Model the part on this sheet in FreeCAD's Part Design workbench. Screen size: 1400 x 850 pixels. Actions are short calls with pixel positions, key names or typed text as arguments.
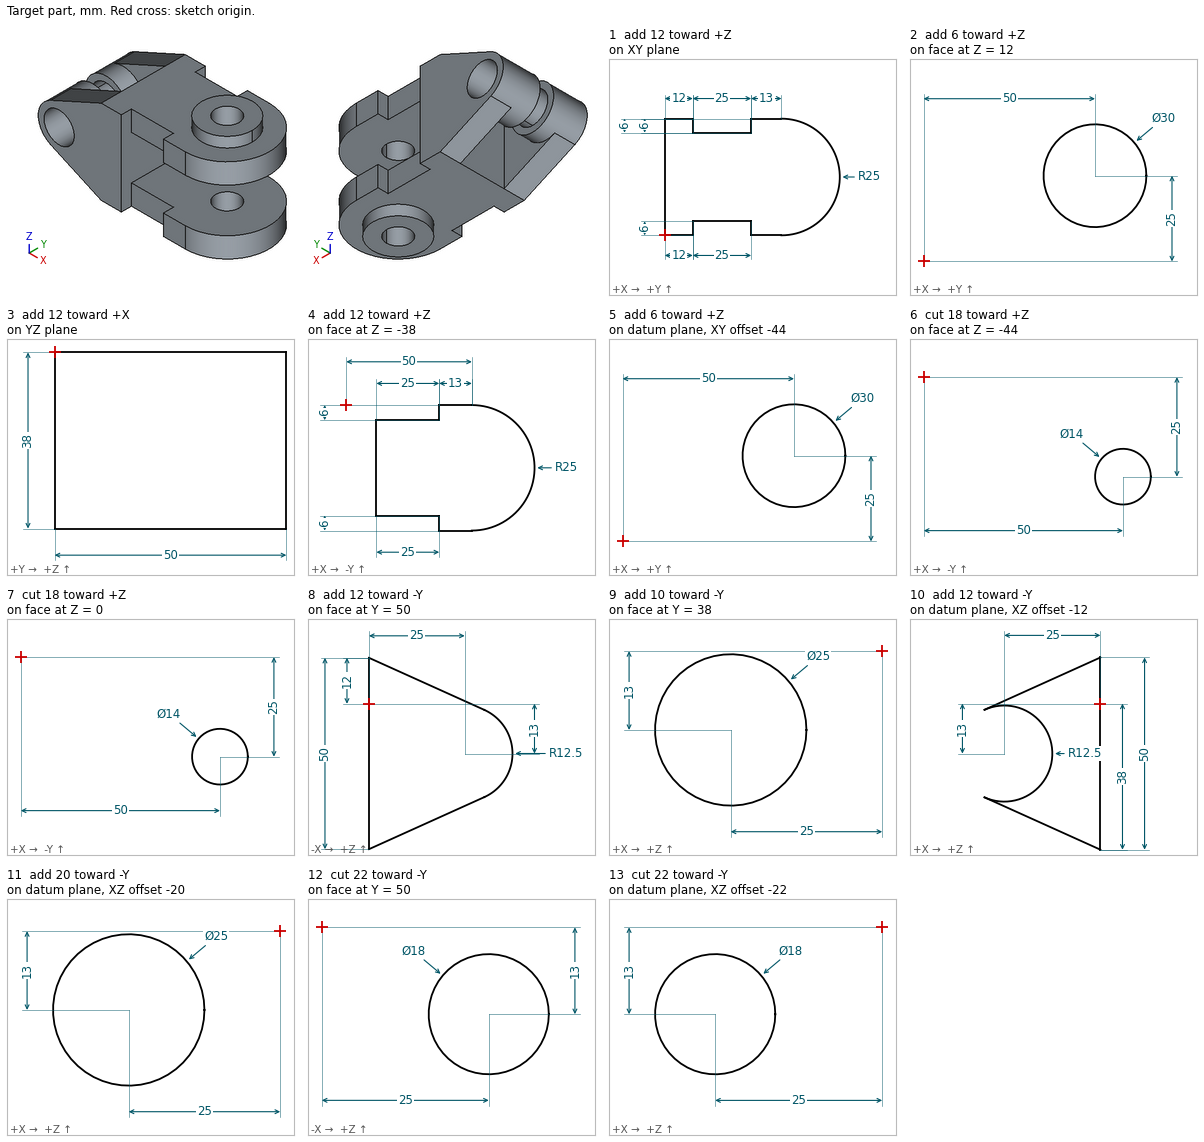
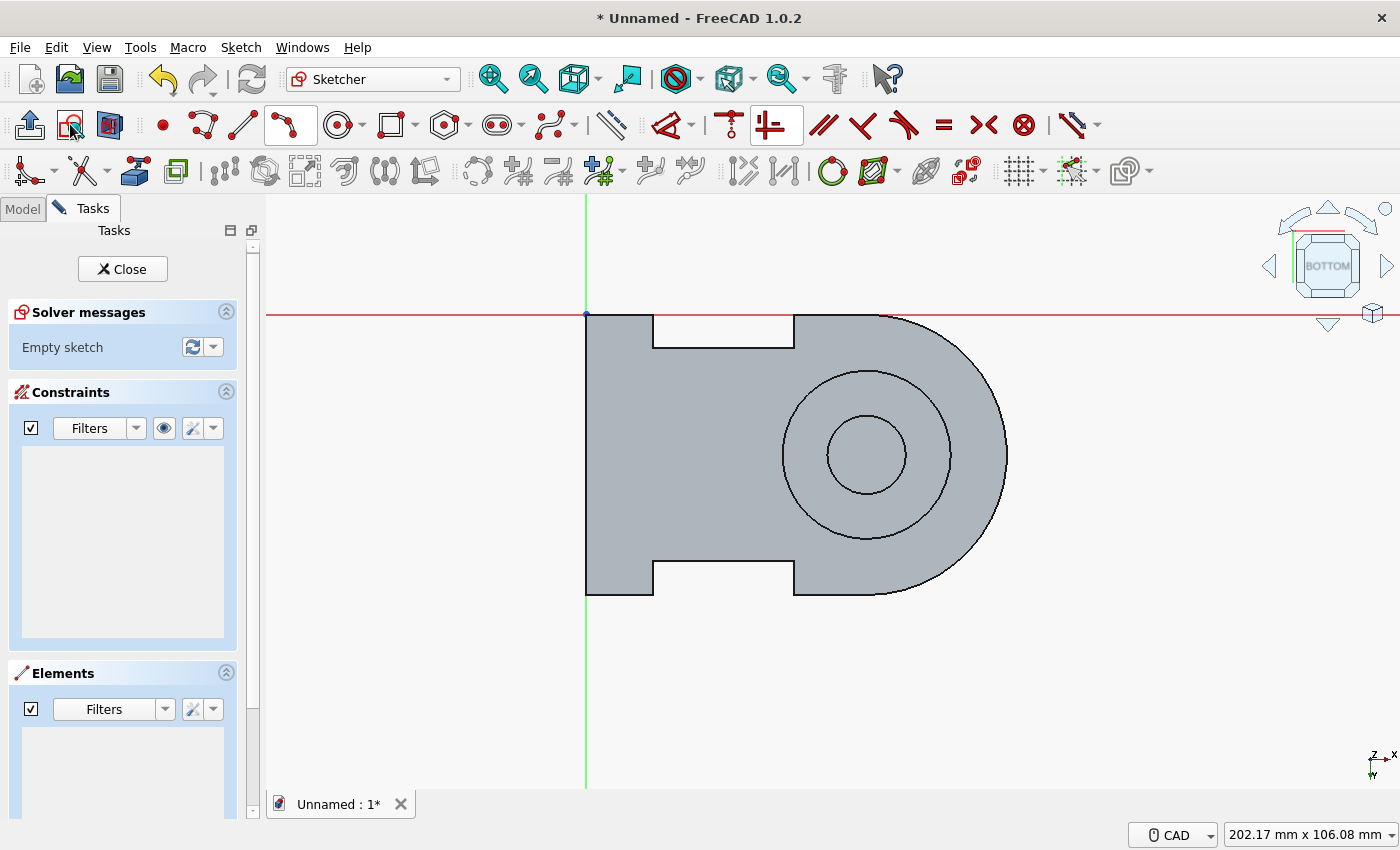
scroll(892, 446, up, 8)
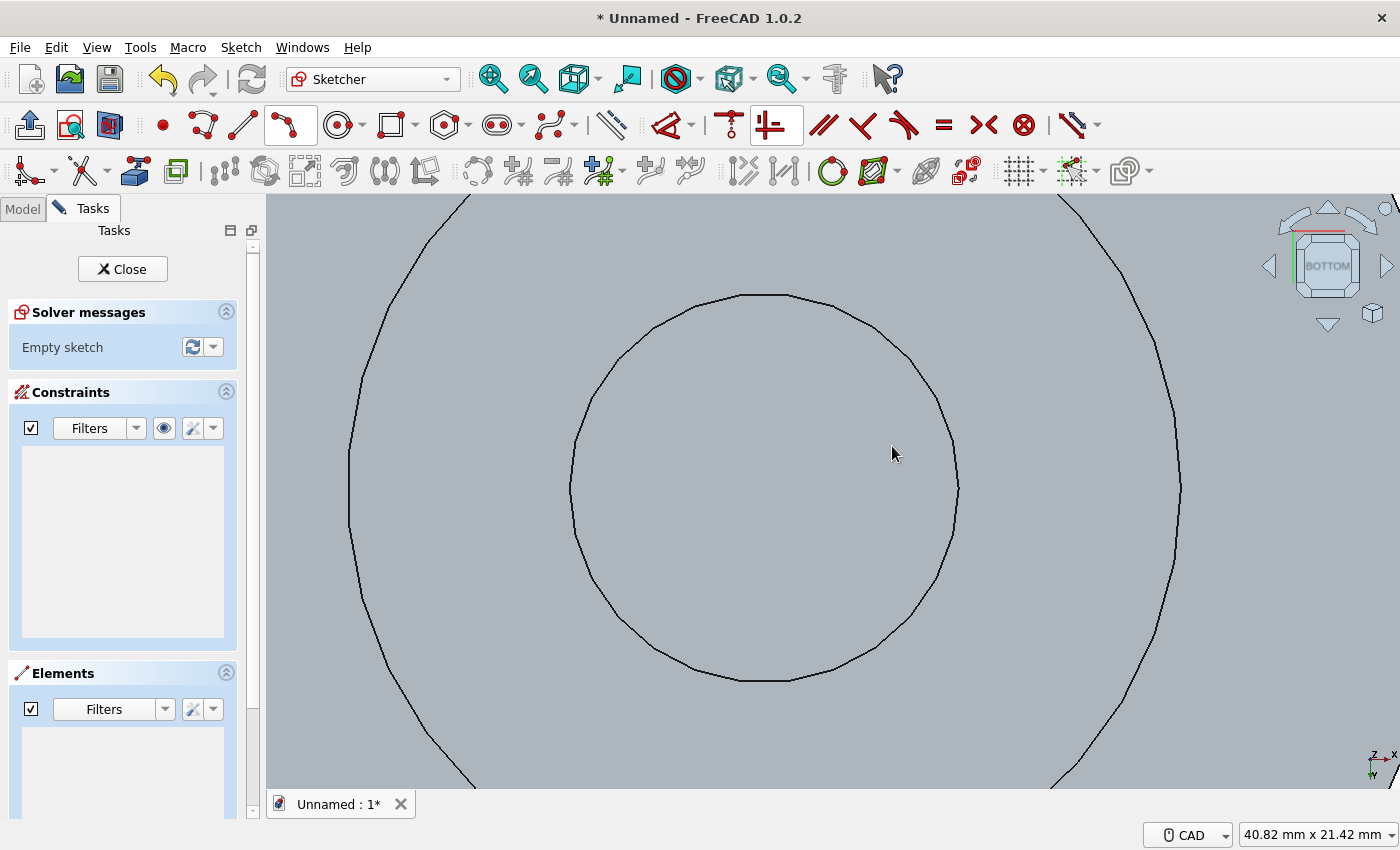
click(338, 126)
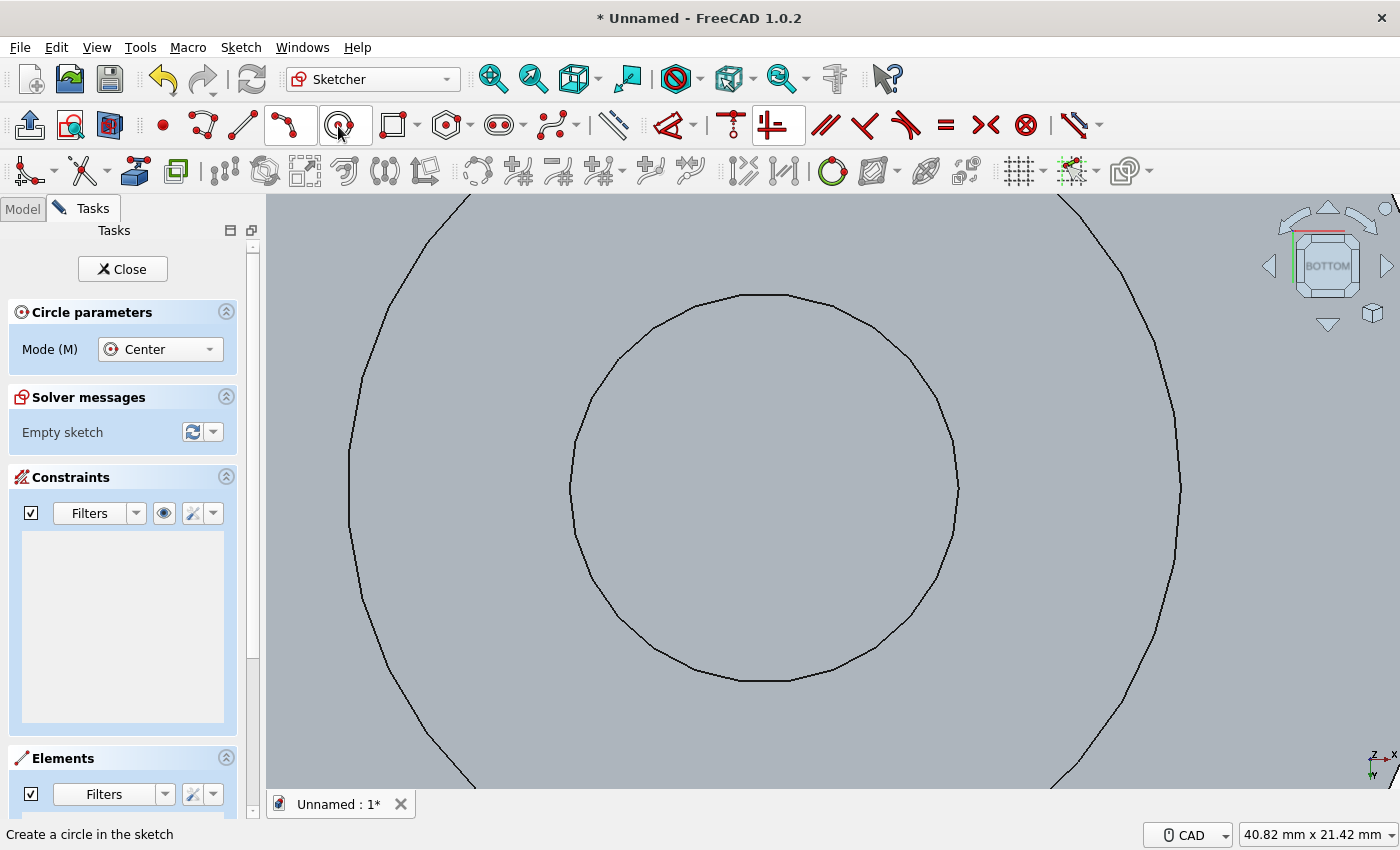
click(764, 488)
click(902, 351)
key(Escape)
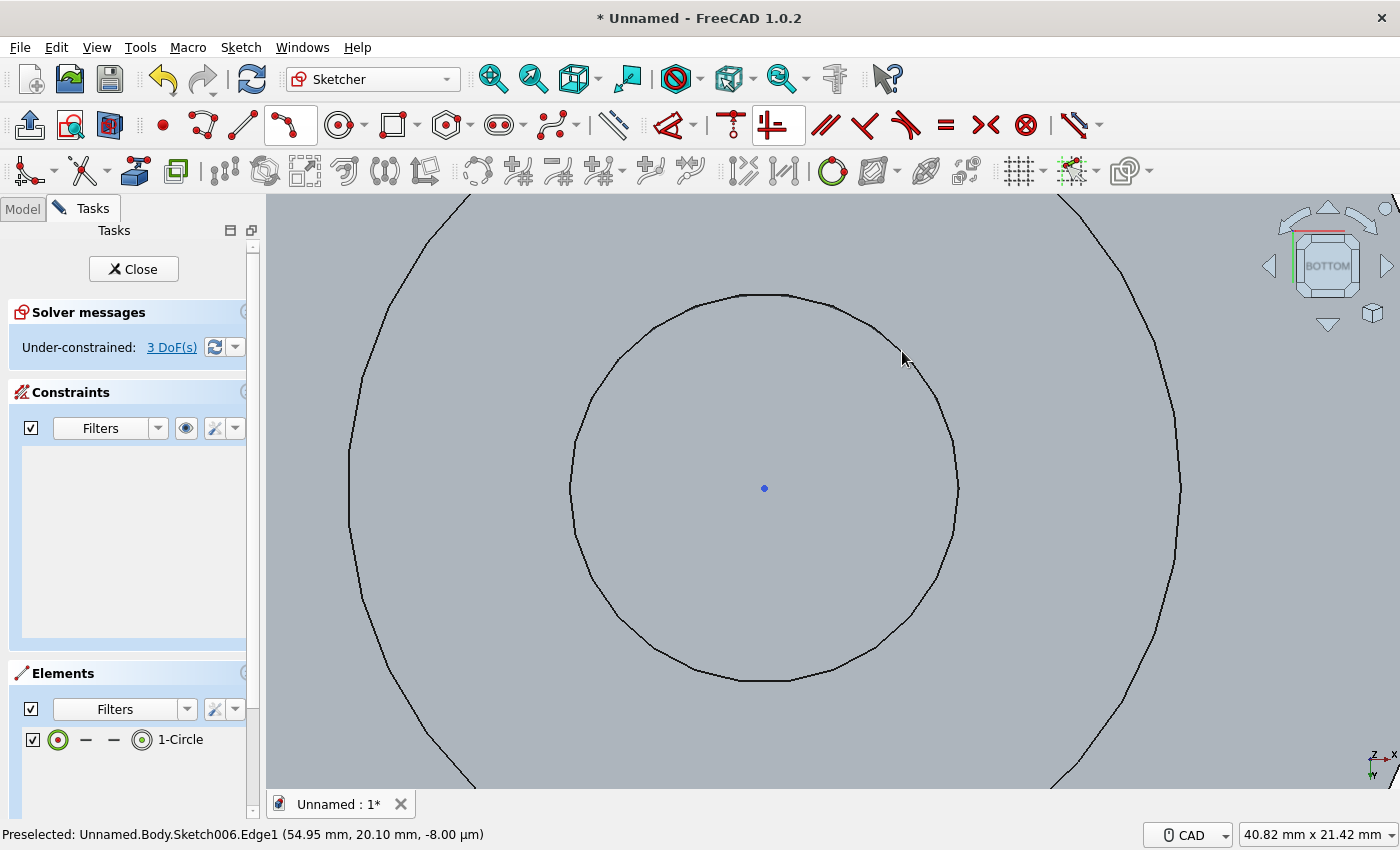
click(668, 126)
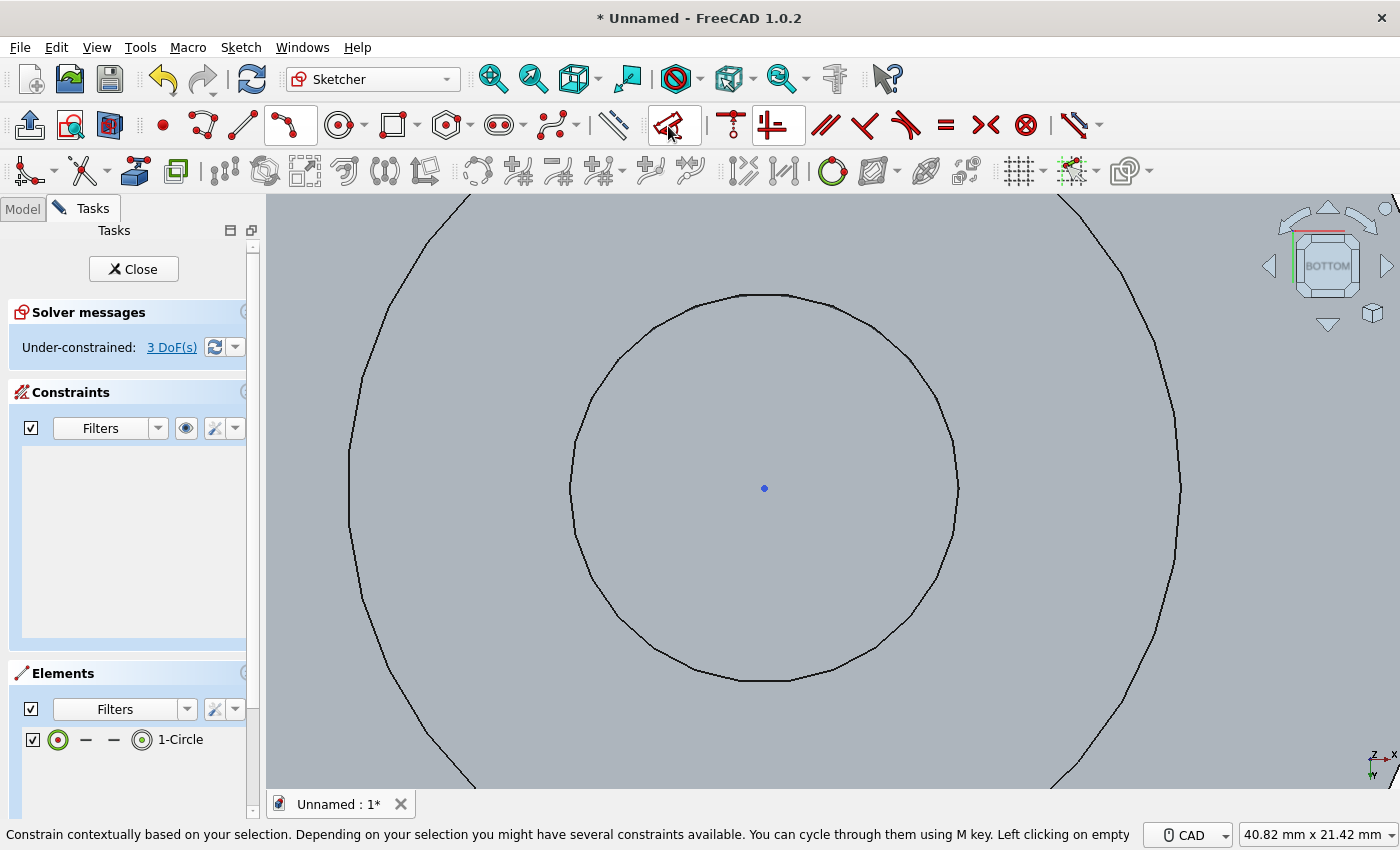
click(901, 351)
click(924, 328)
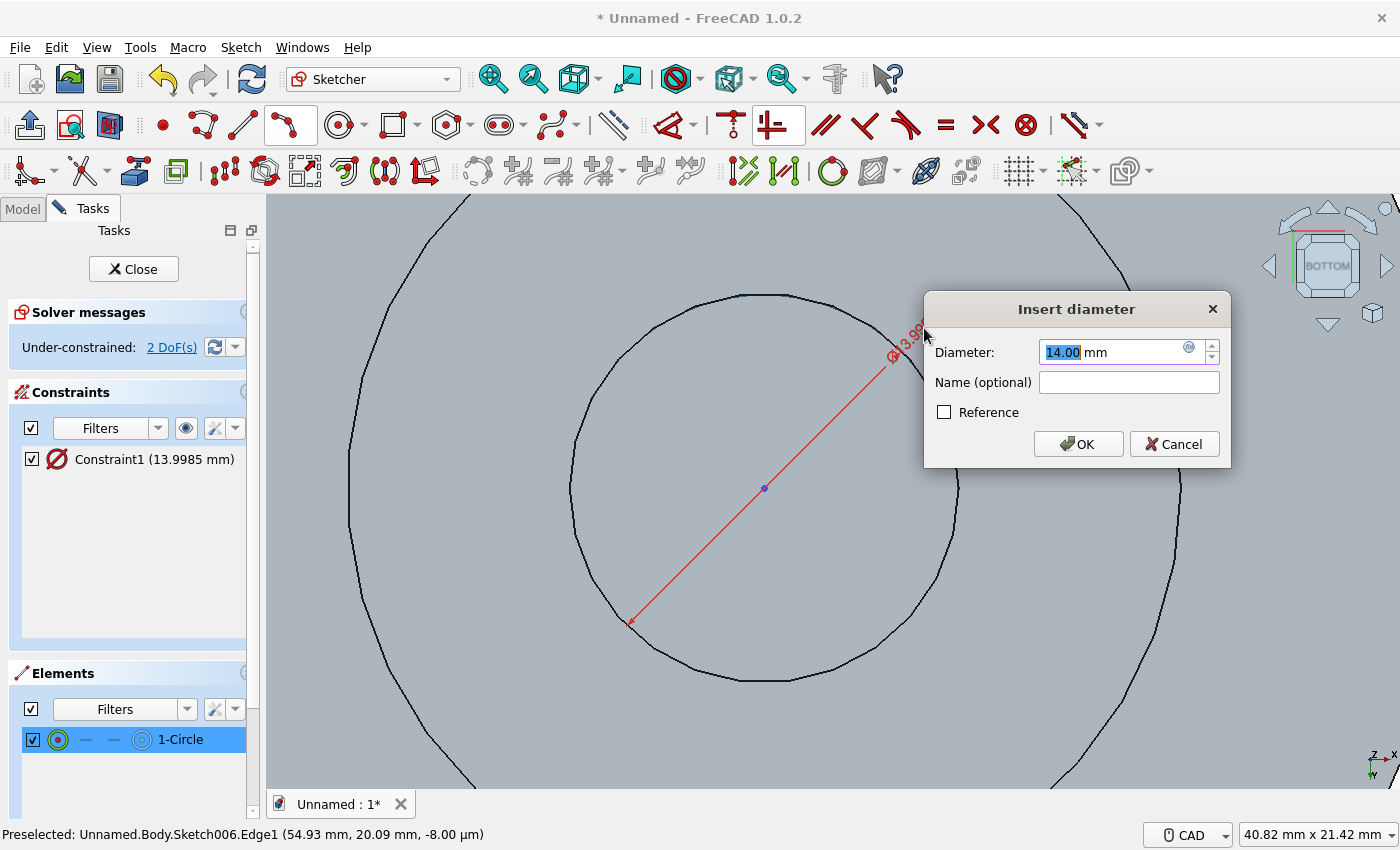
text(14)
key(Return)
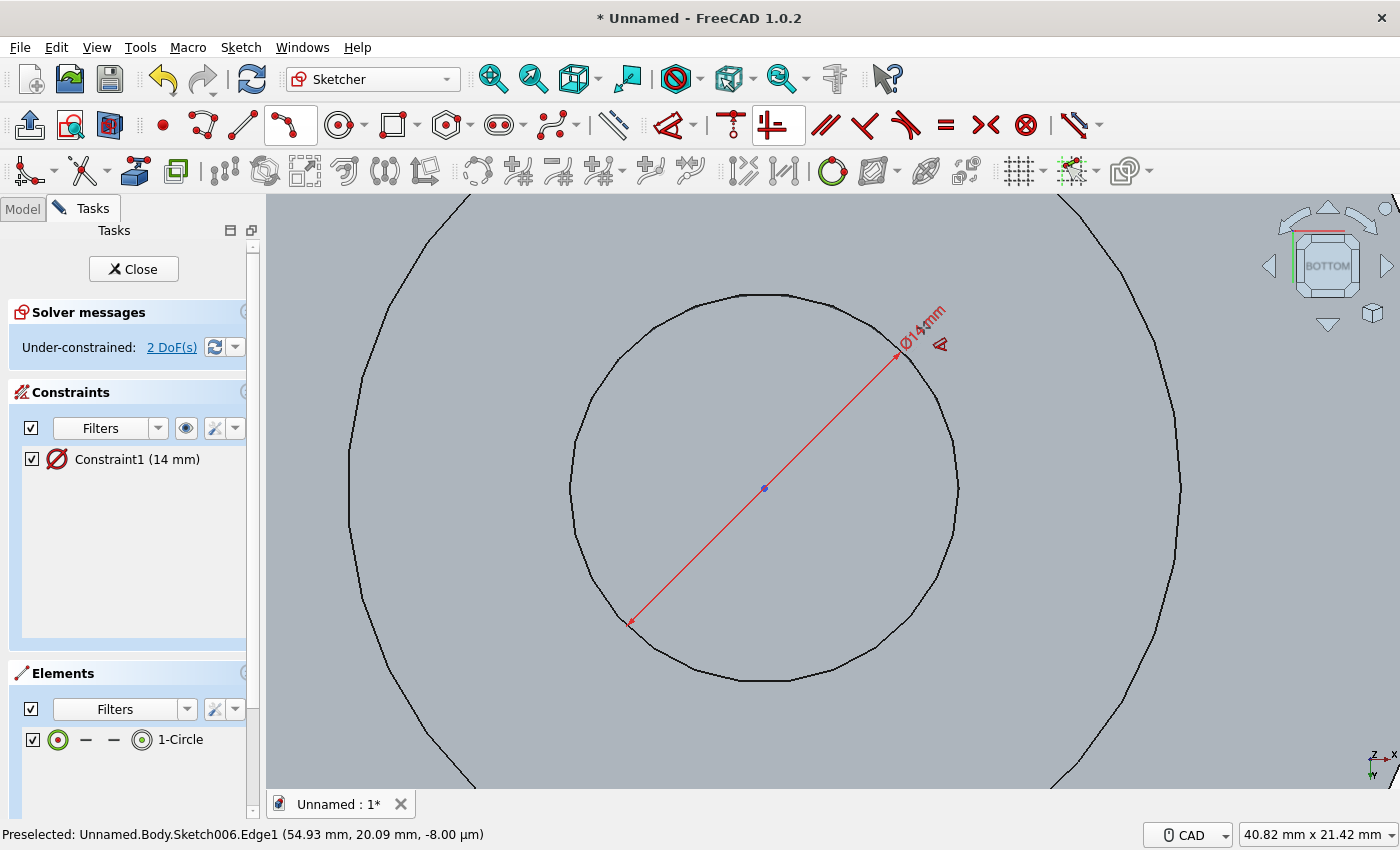
click(764, 489)
click(529, 523)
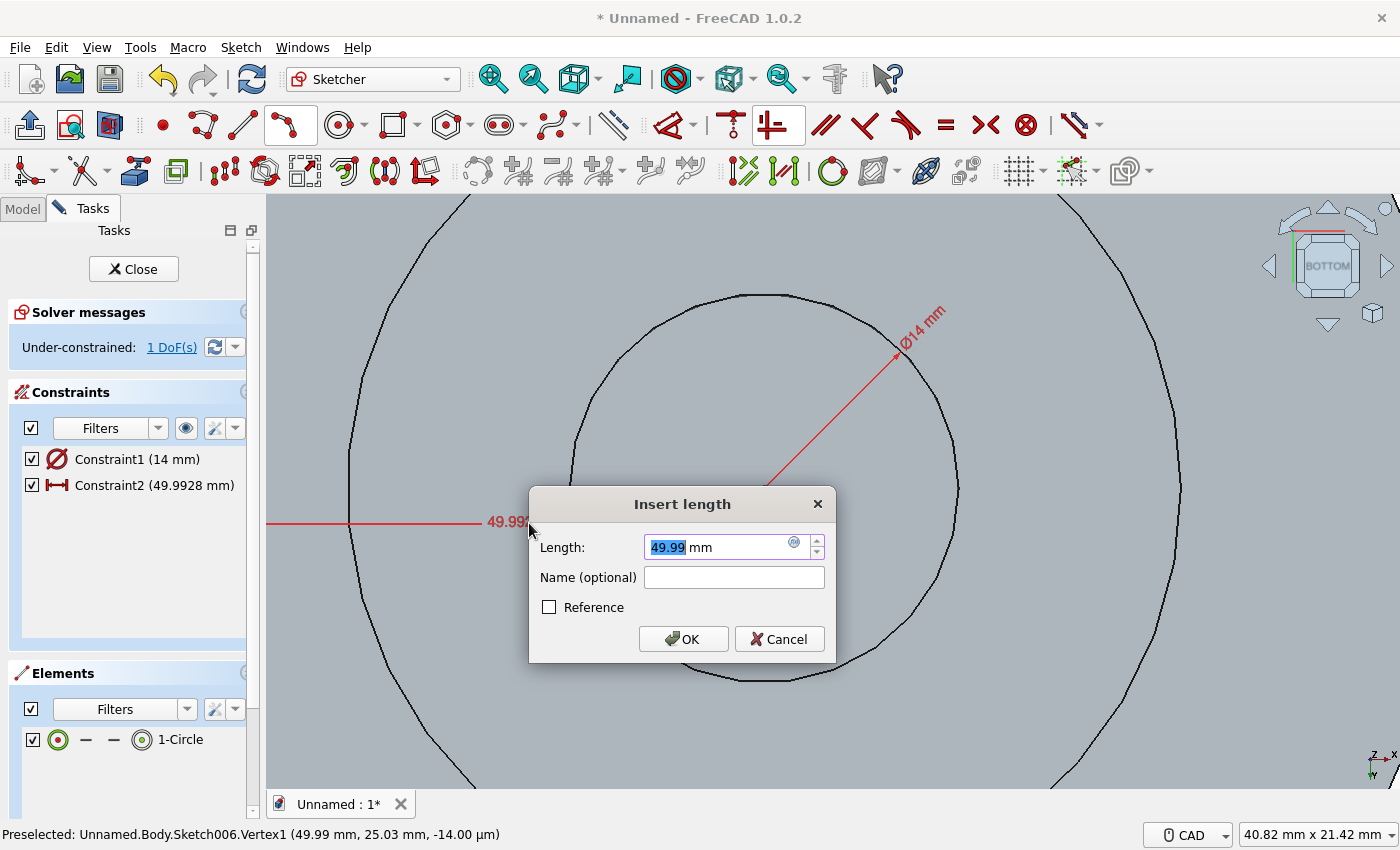
text(50)
key(Return)